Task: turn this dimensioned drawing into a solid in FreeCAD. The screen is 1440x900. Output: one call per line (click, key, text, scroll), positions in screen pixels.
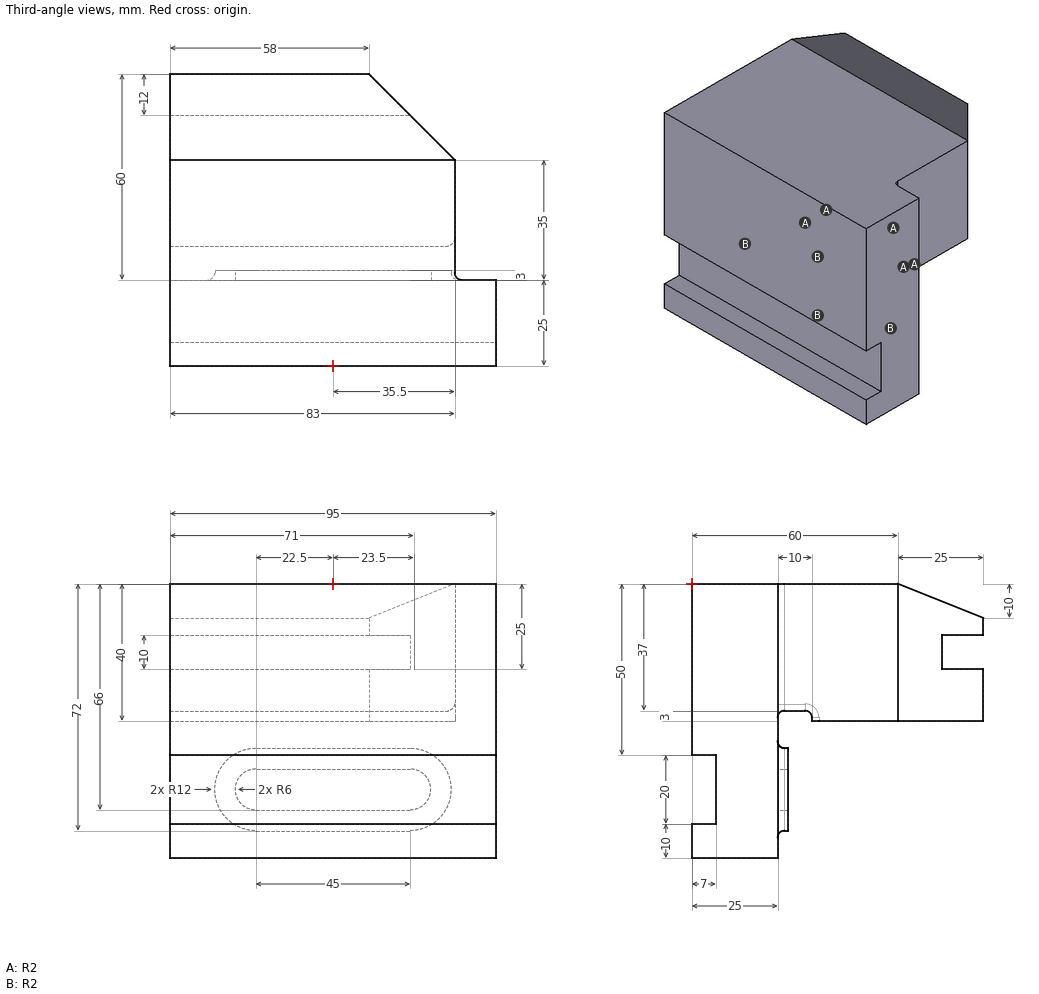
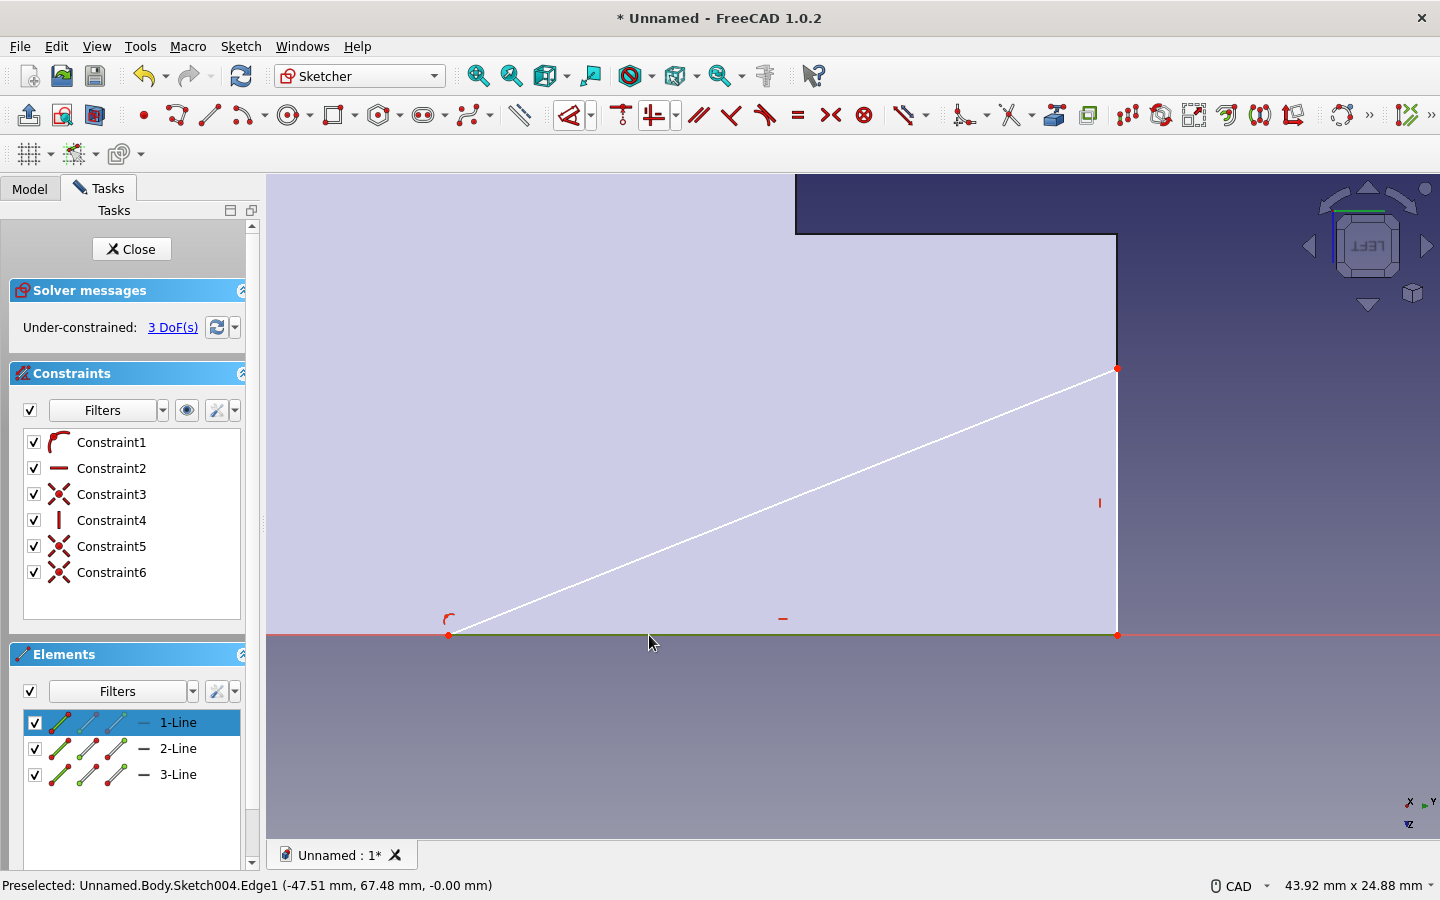
click(590, 116)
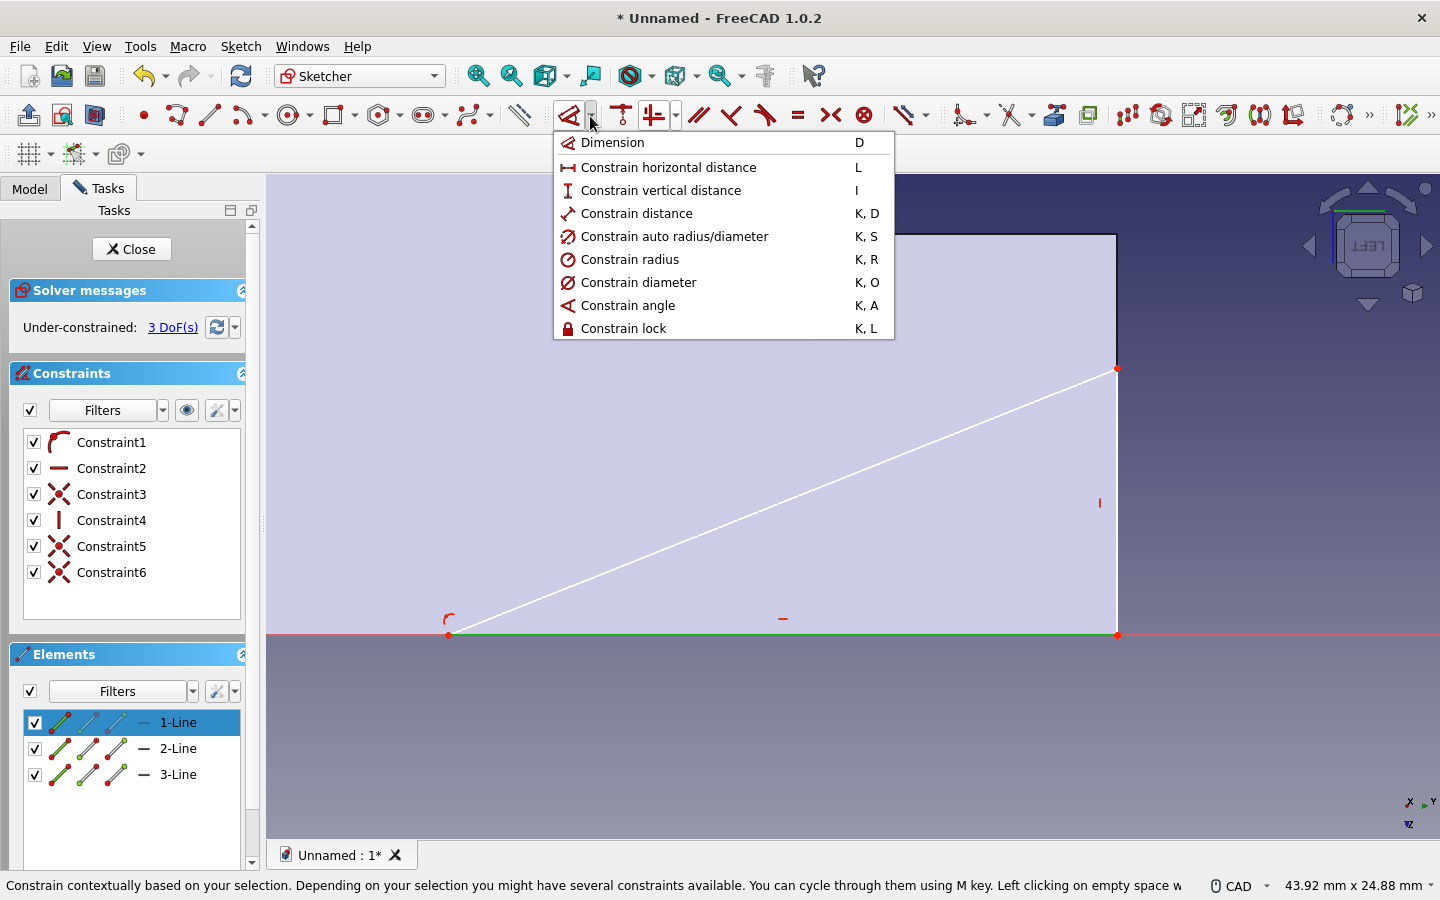
click(724, 168)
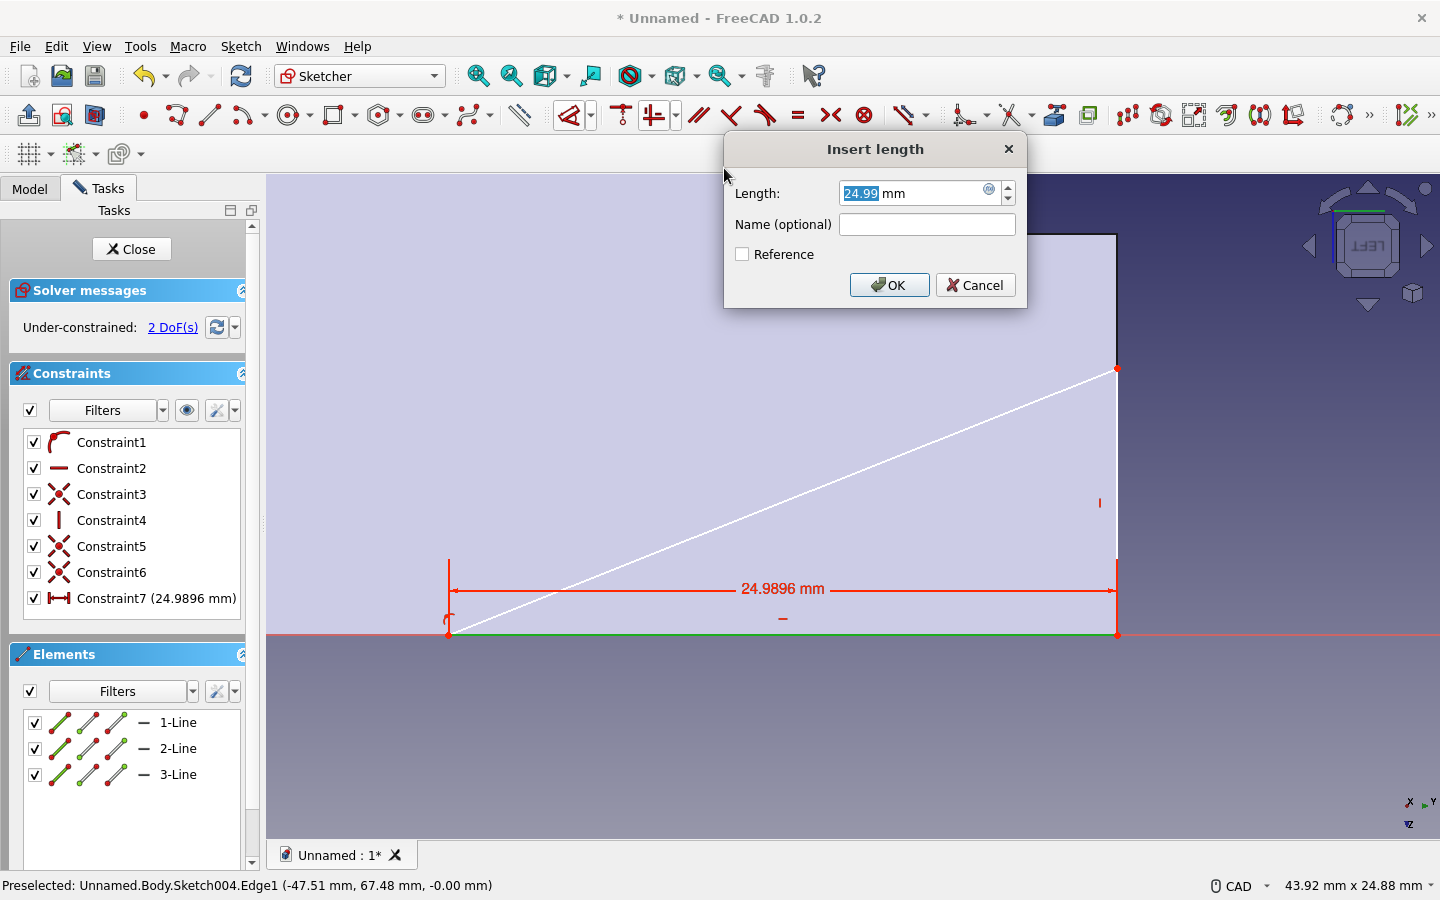
text(25)
key(Return)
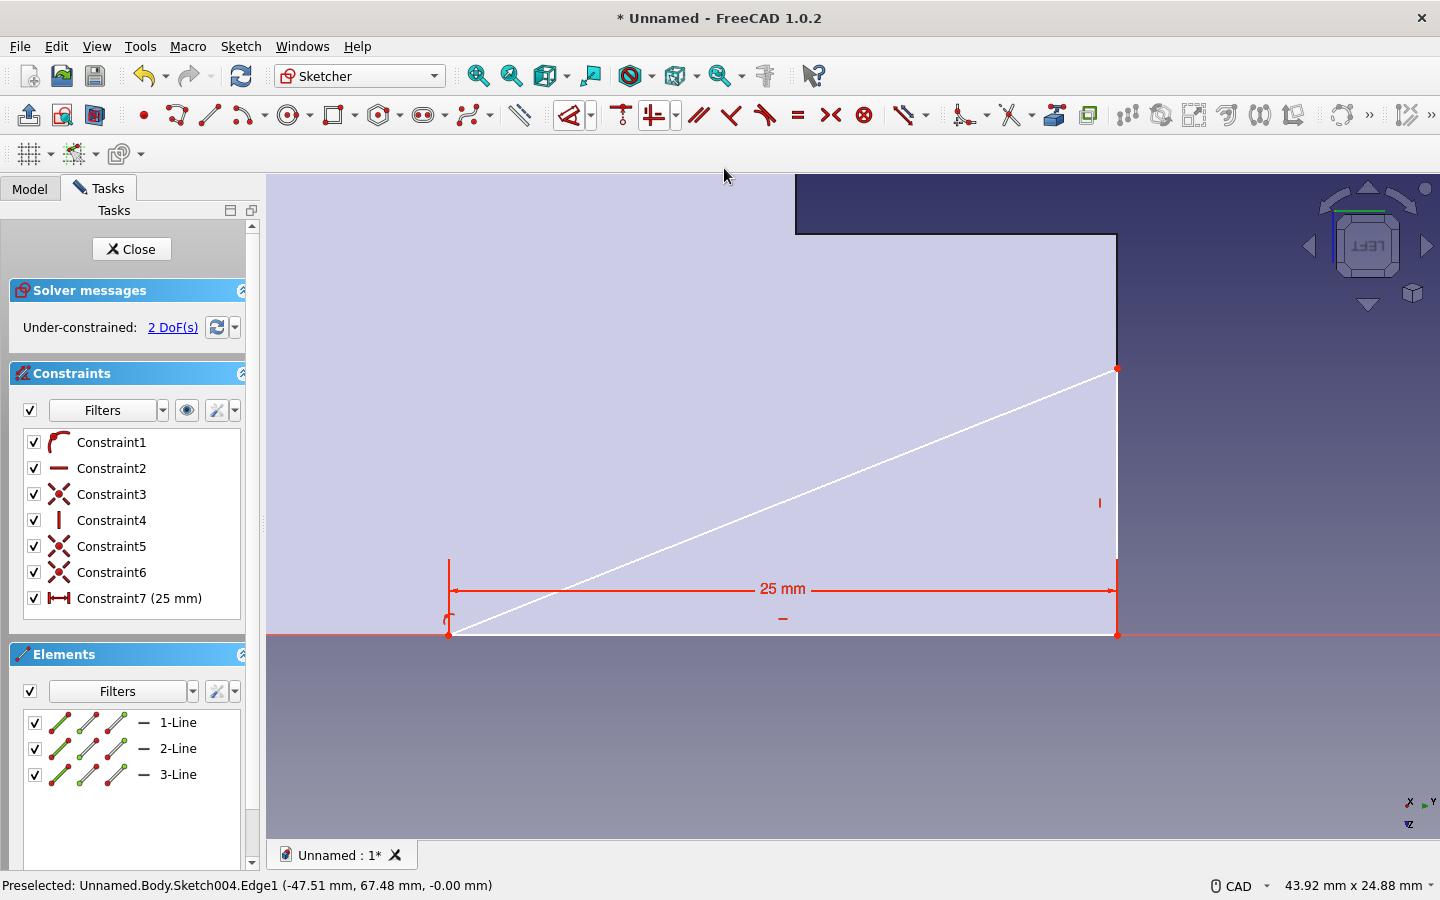
click(1117, 555)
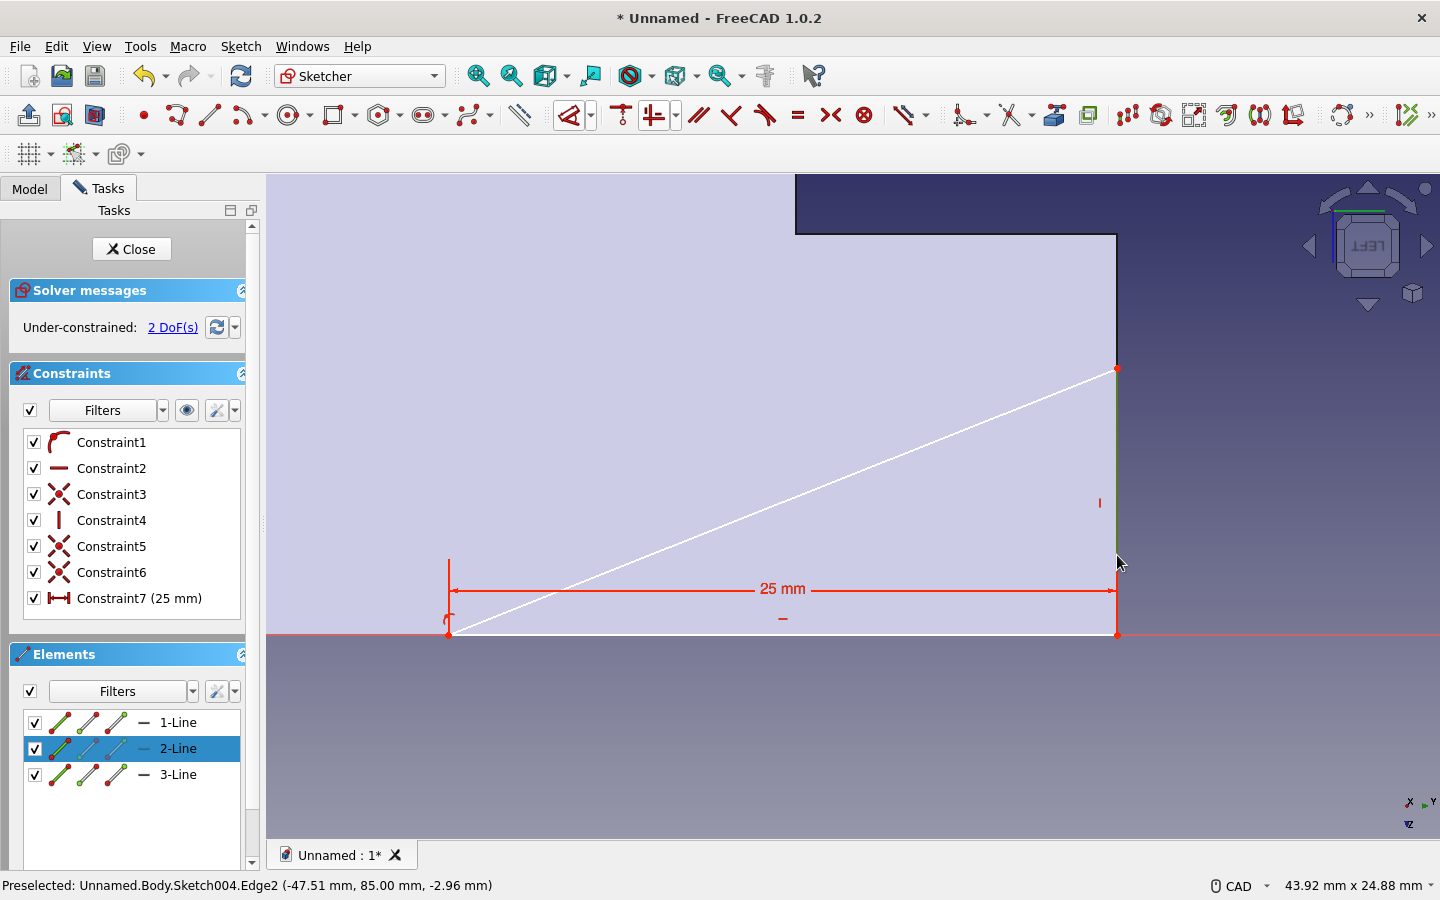
click(590, 116)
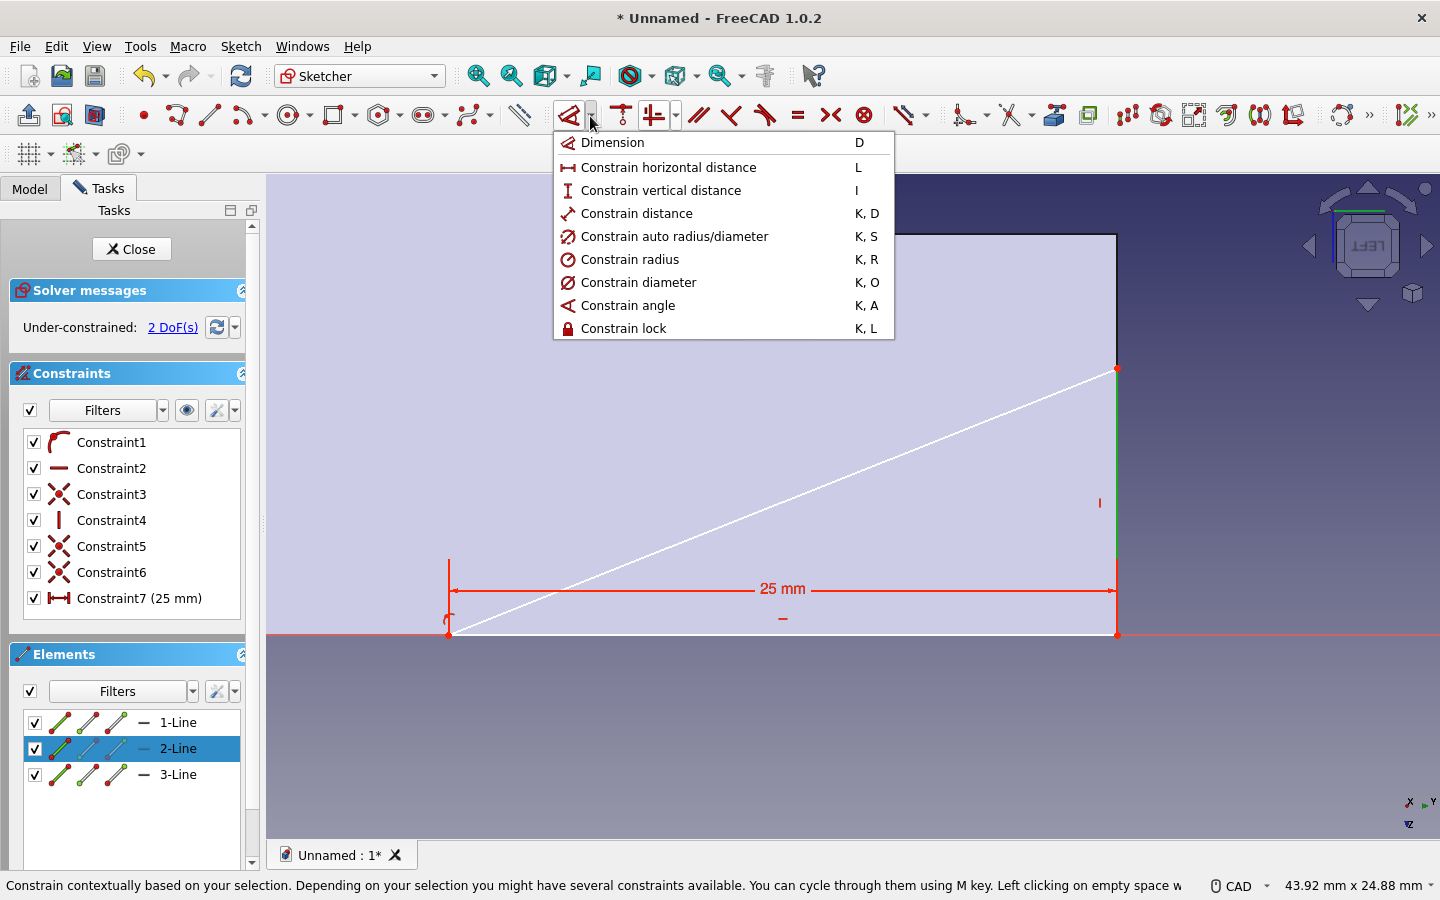
click(724, 190)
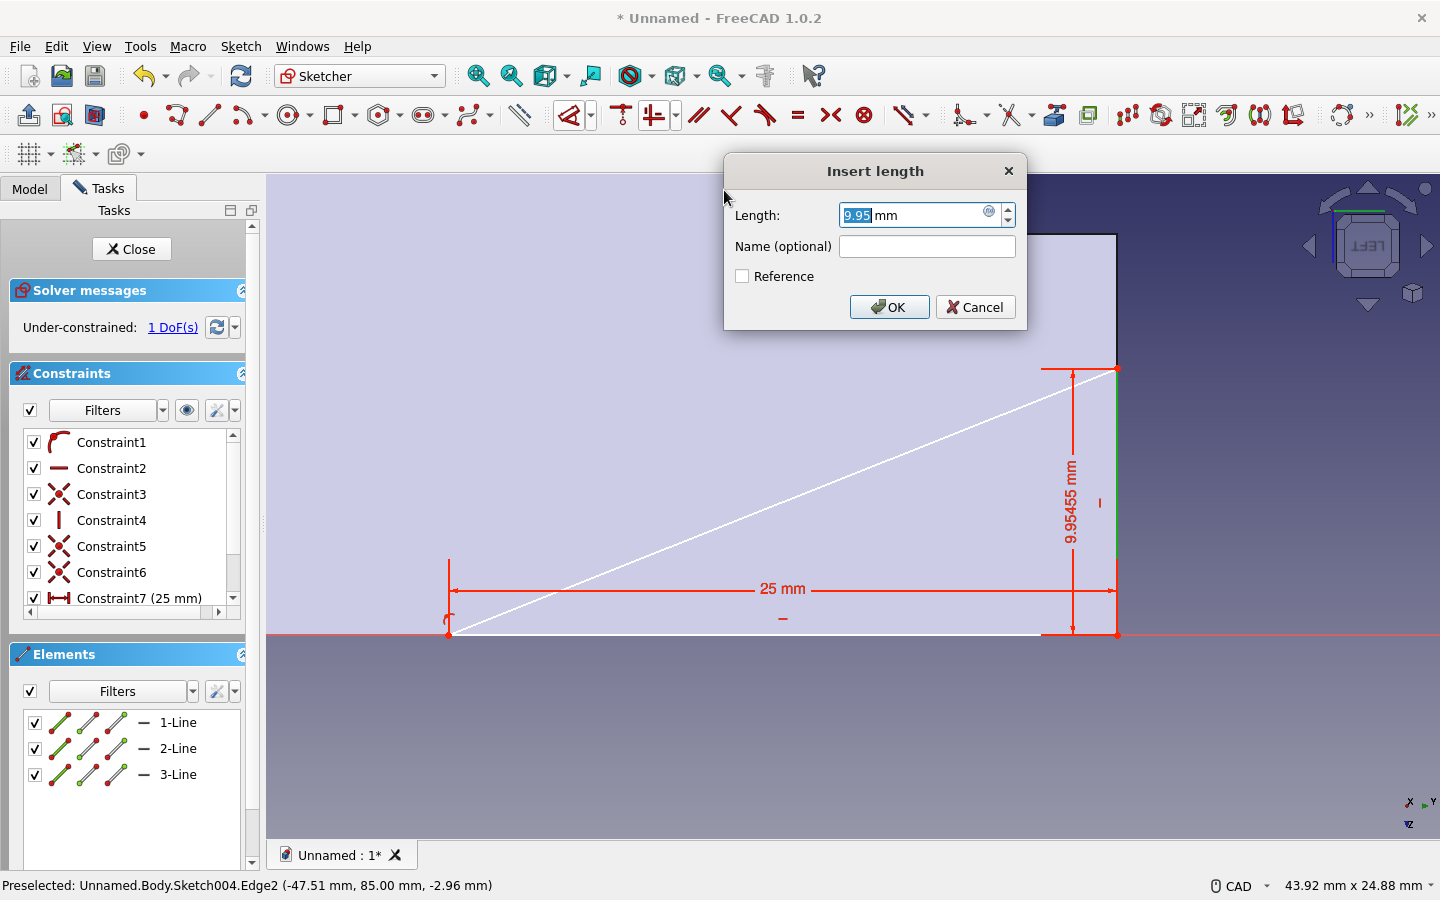
text(10)
key(Return)